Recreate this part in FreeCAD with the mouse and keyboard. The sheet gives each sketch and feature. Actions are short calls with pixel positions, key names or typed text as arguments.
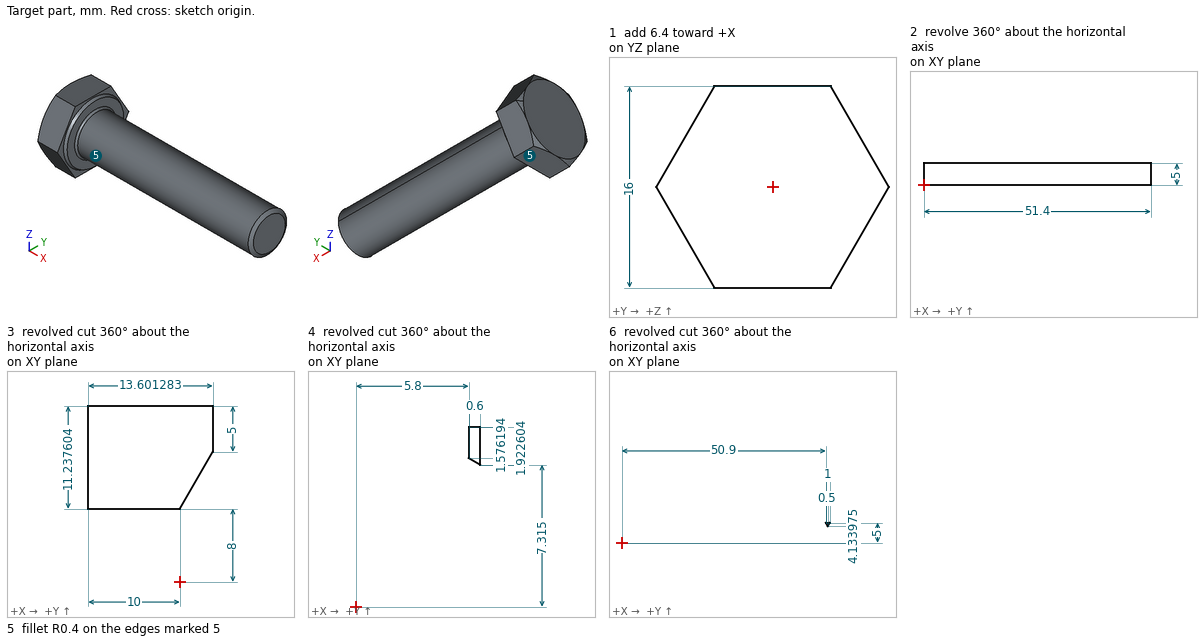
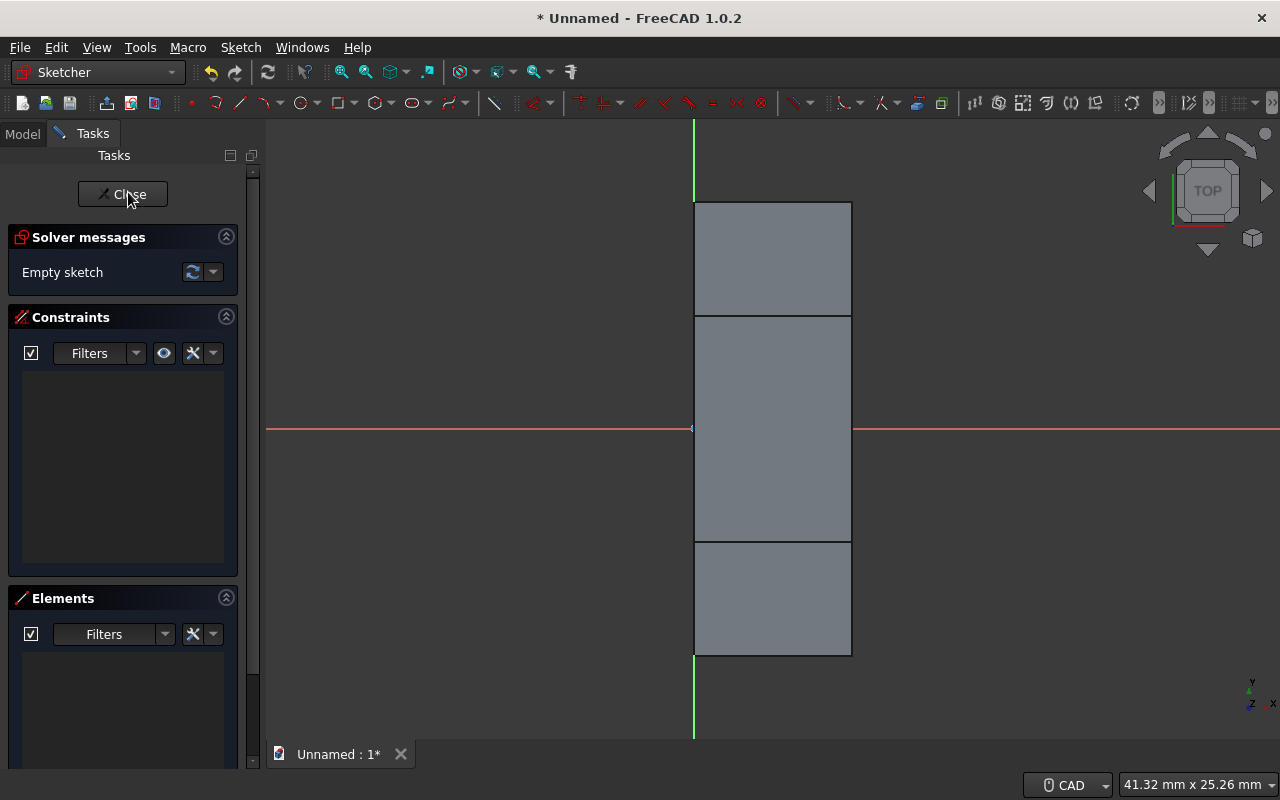
click(156, 104)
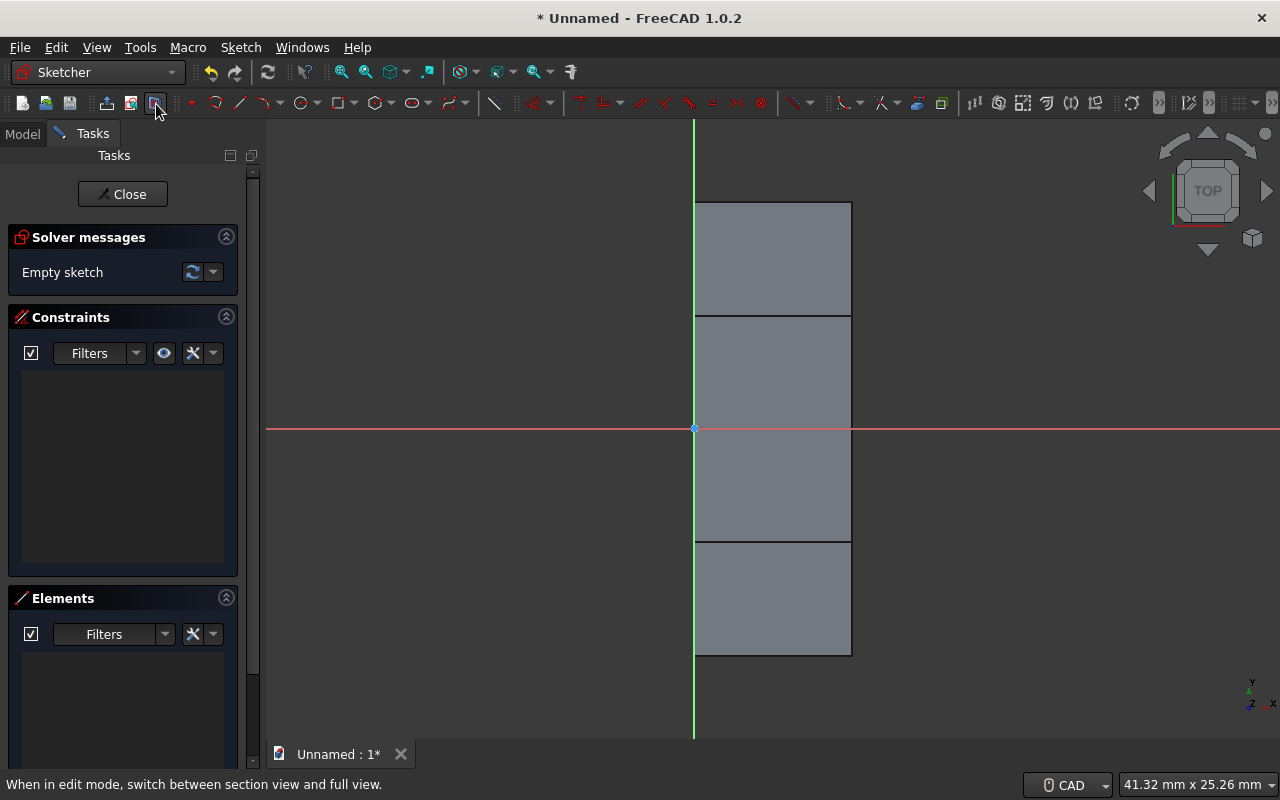
scroll(294, 479, down, 4)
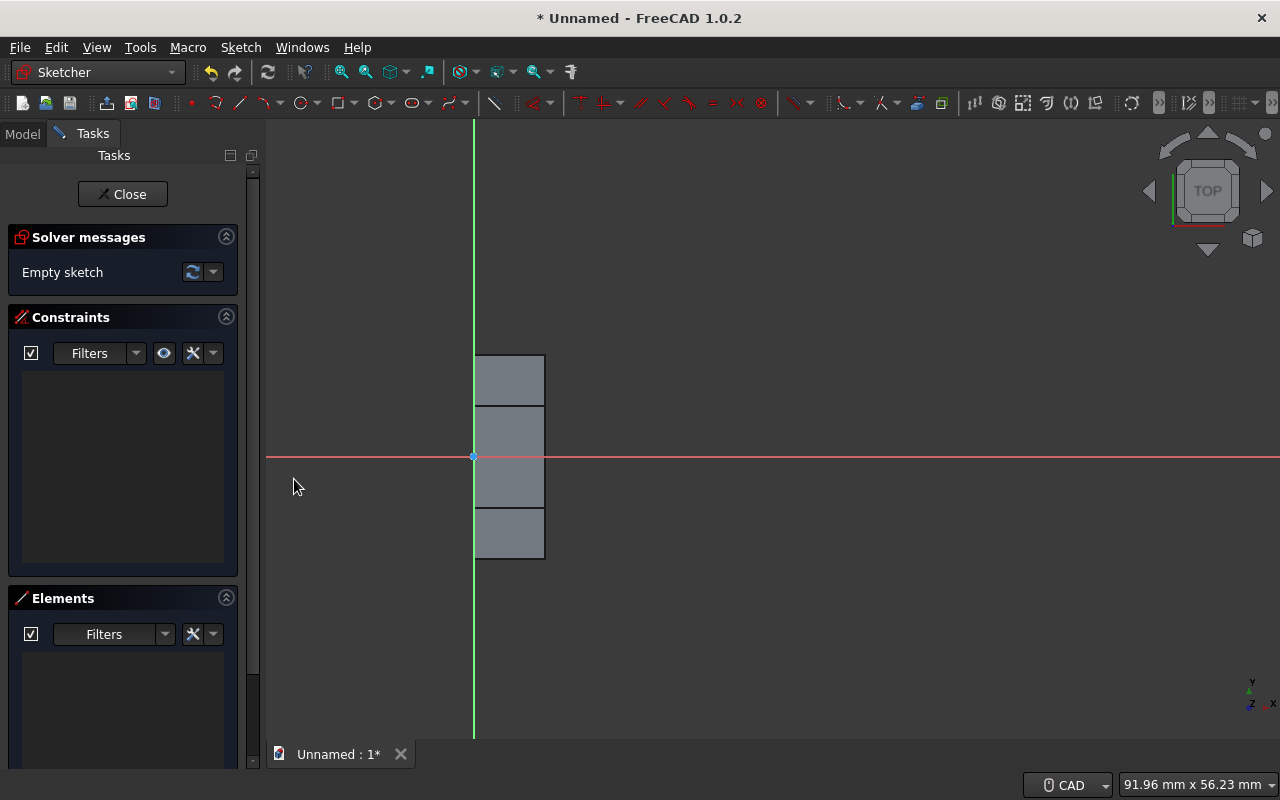
click(338, 104)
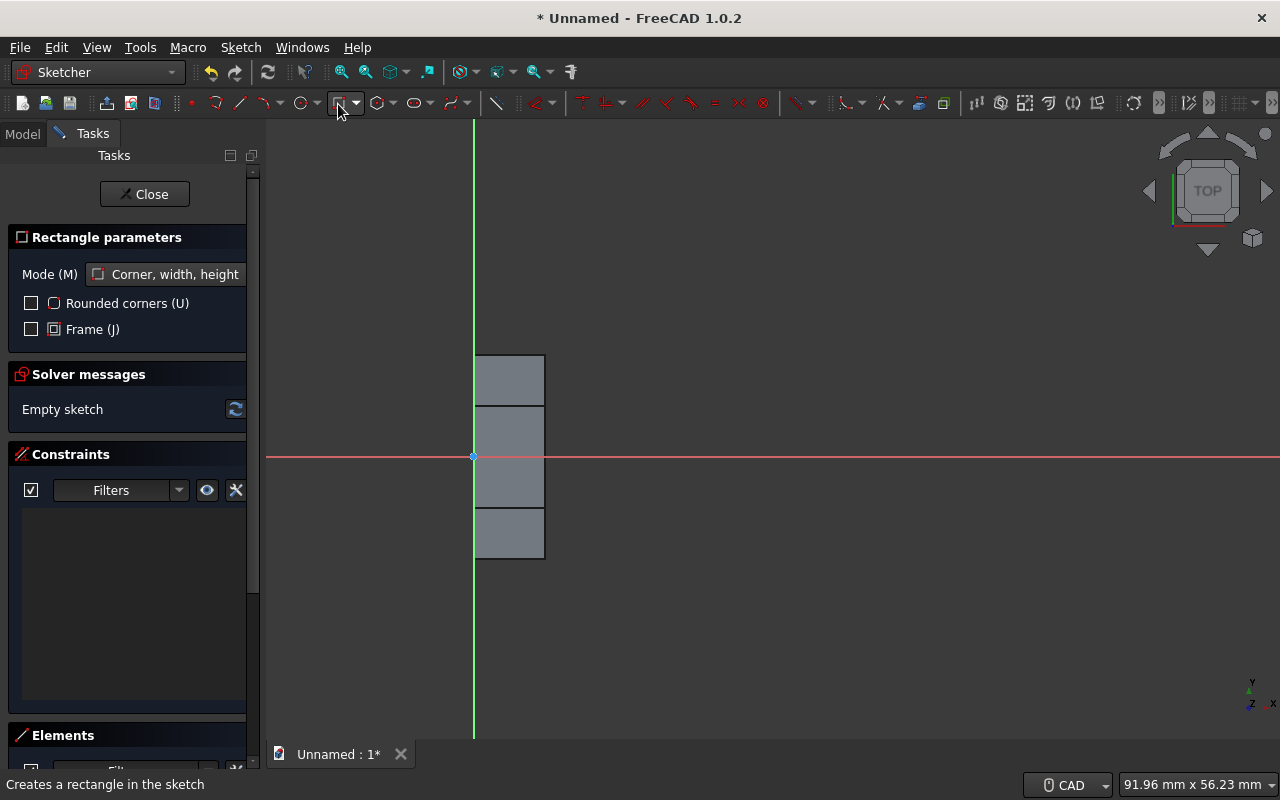
click(474, 457)
click(1041, 402)
key(Escape)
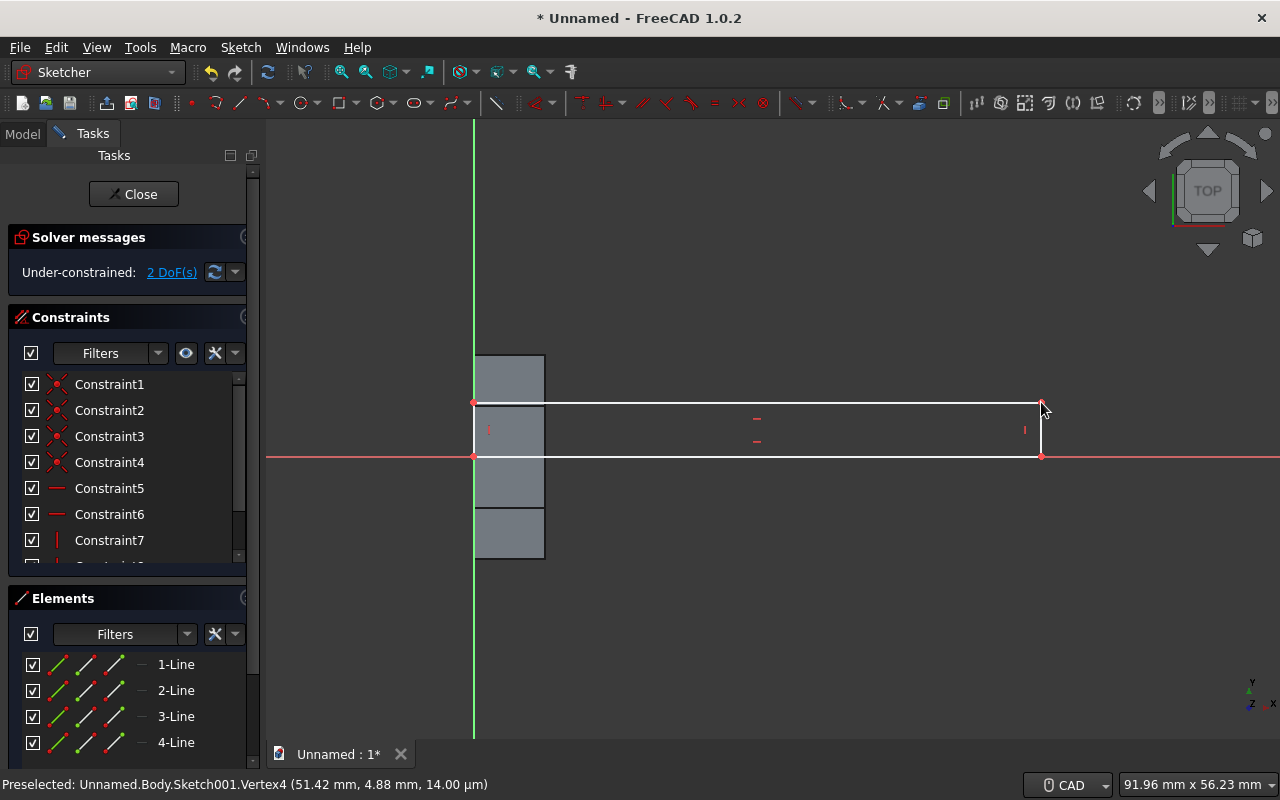
click(536, 104)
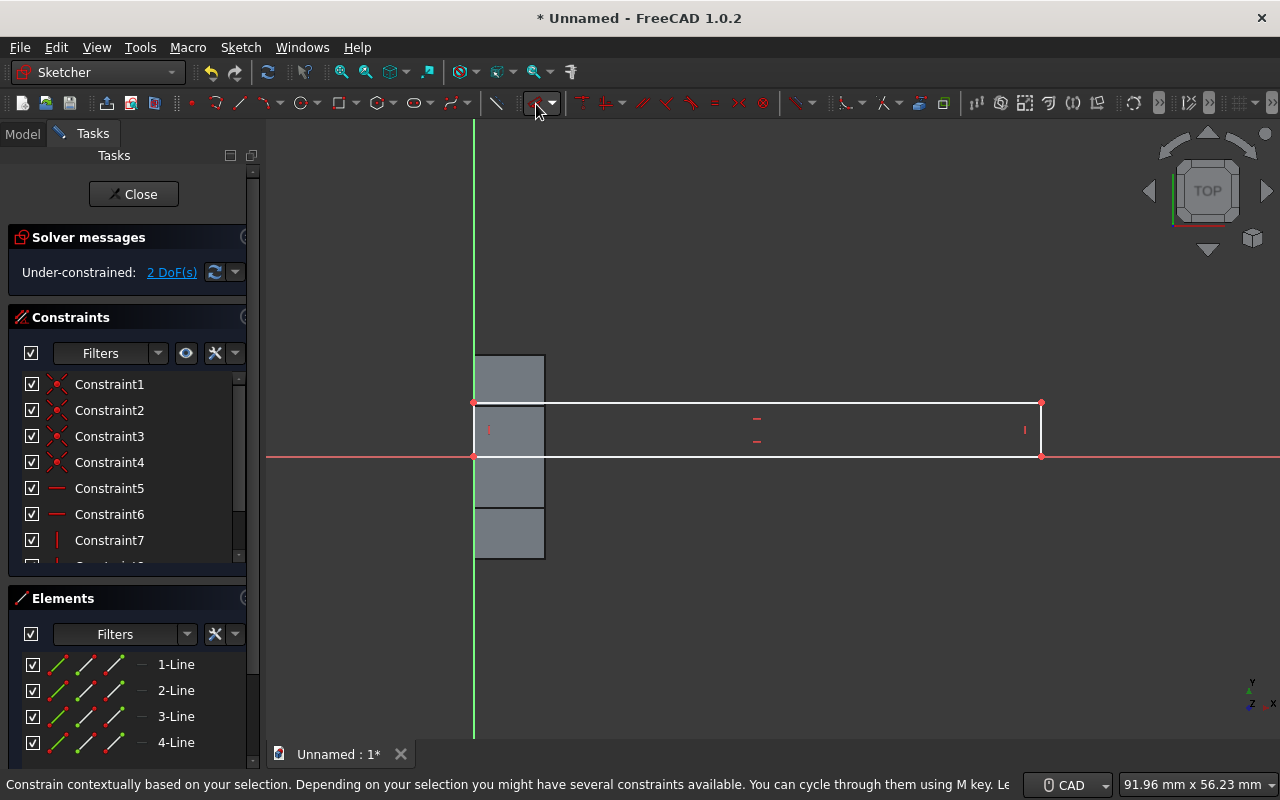
click(1041, 441)
click(1075, 430)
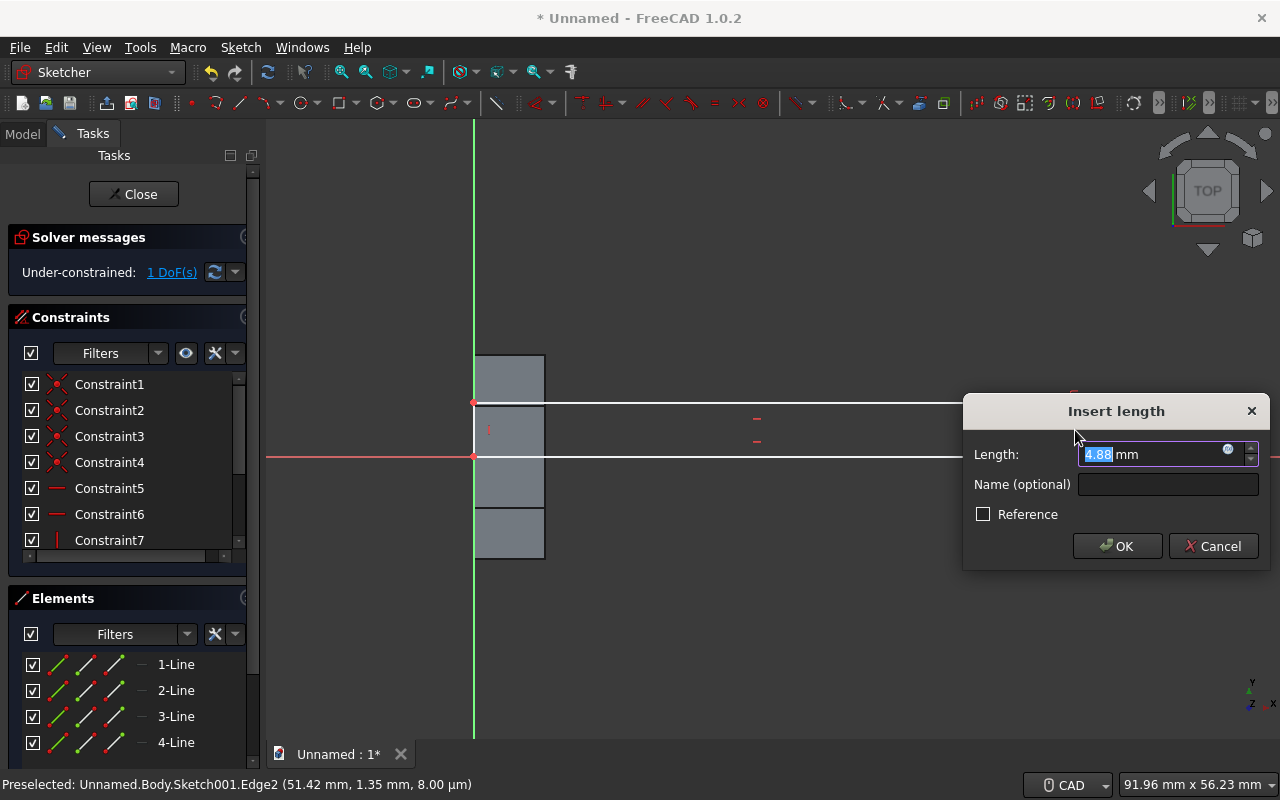
text(5)
key(Return)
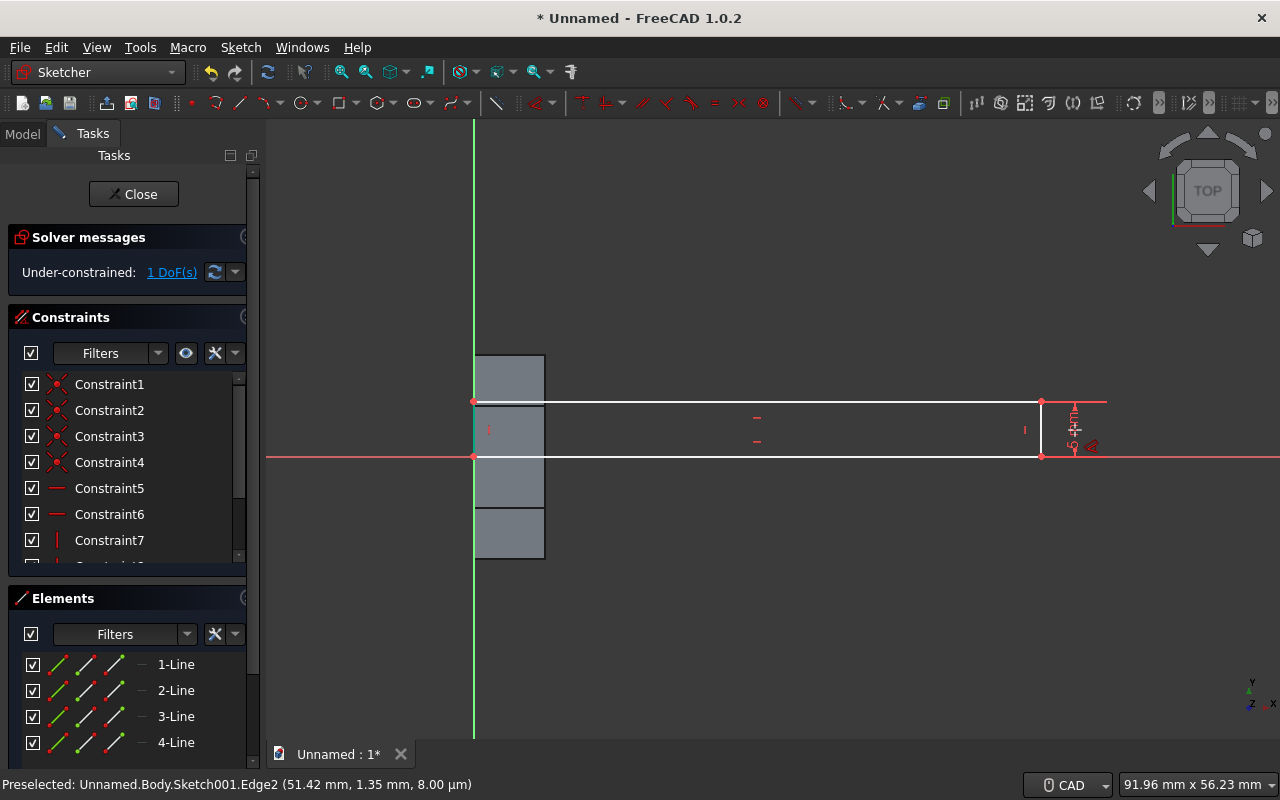
click(644, 457)
click(757, 491)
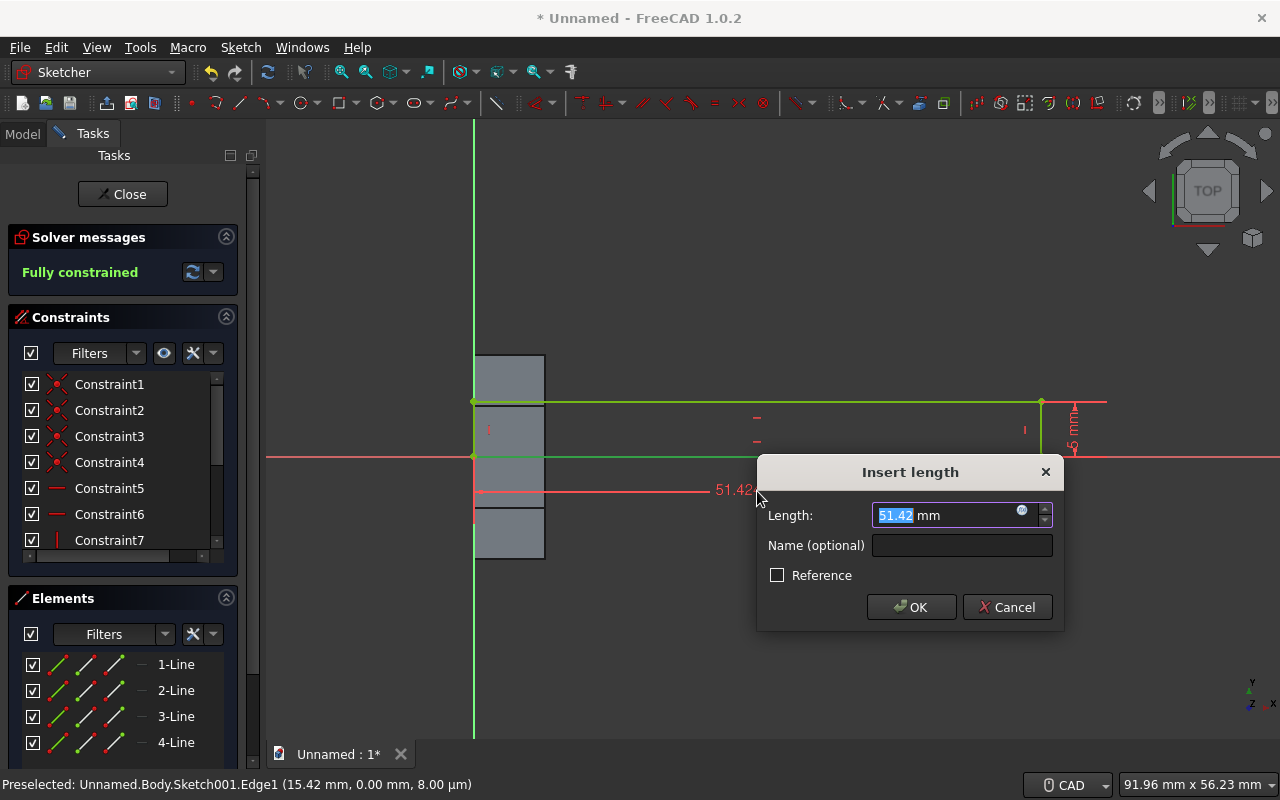
text(51.4)
key(Return)
key(Escape)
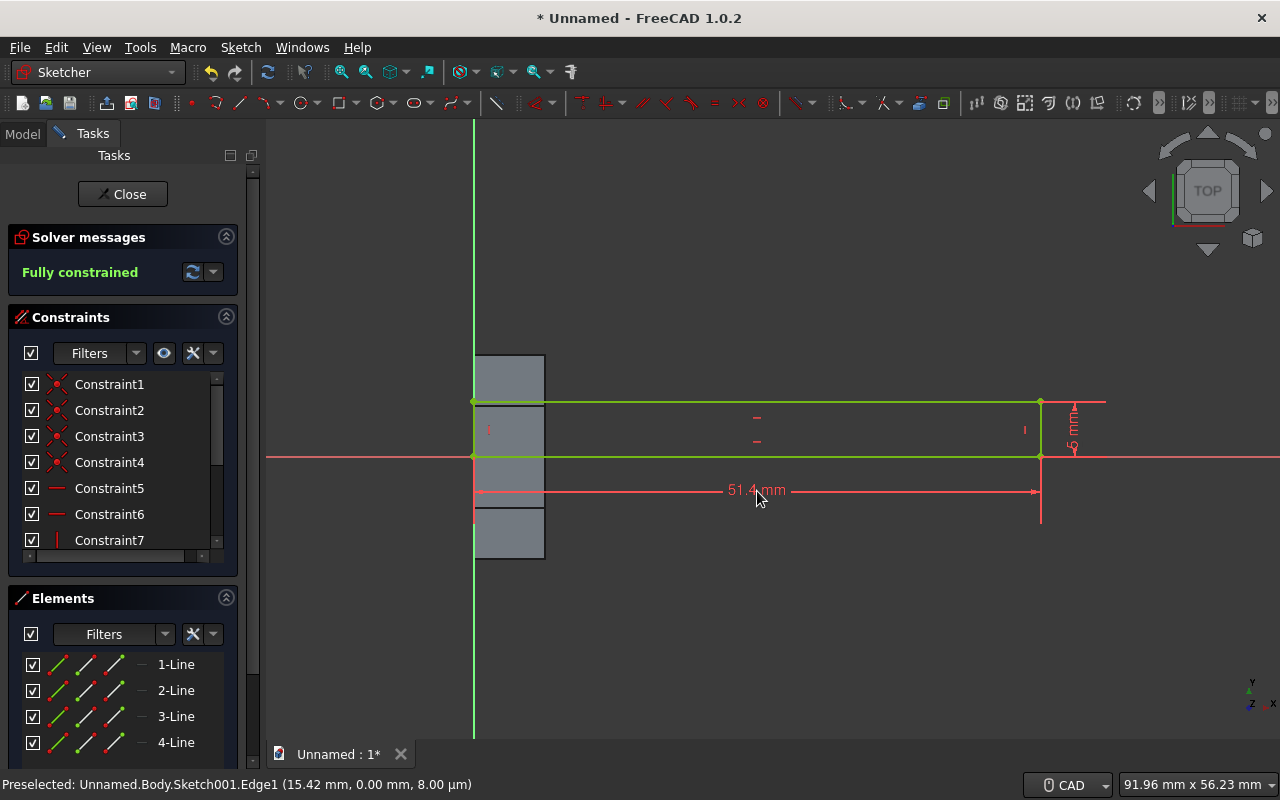
click(123, 194)